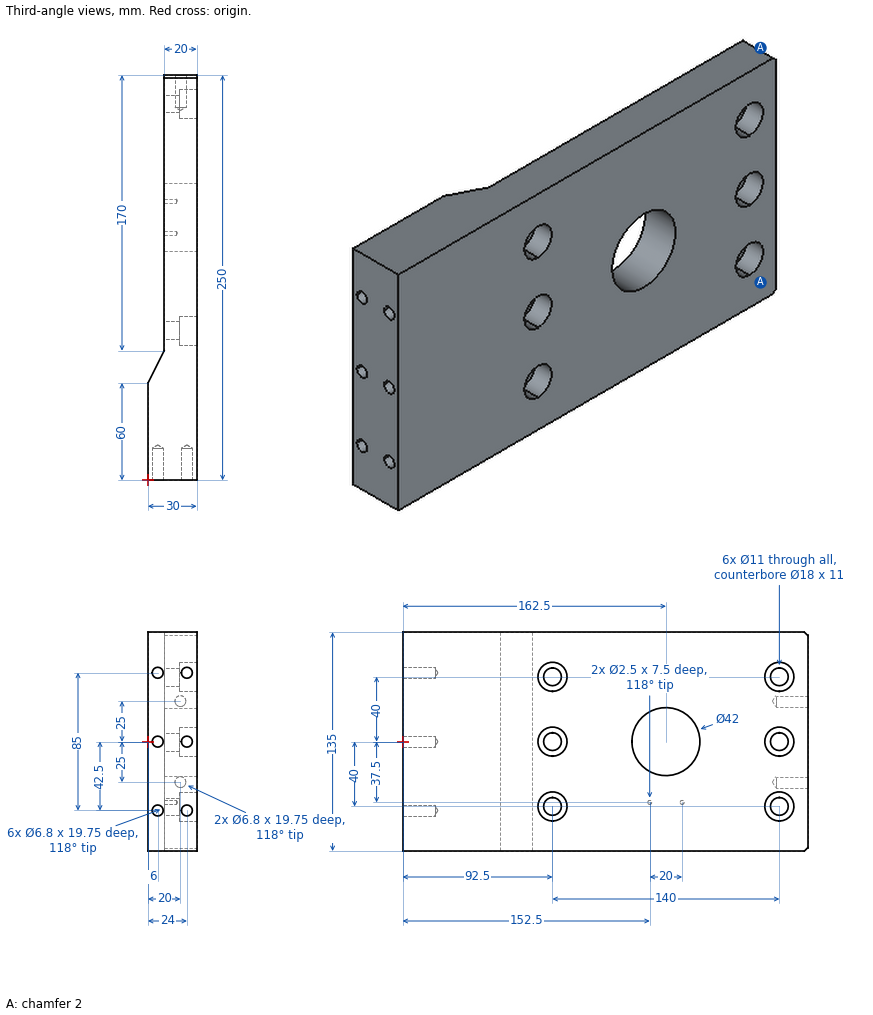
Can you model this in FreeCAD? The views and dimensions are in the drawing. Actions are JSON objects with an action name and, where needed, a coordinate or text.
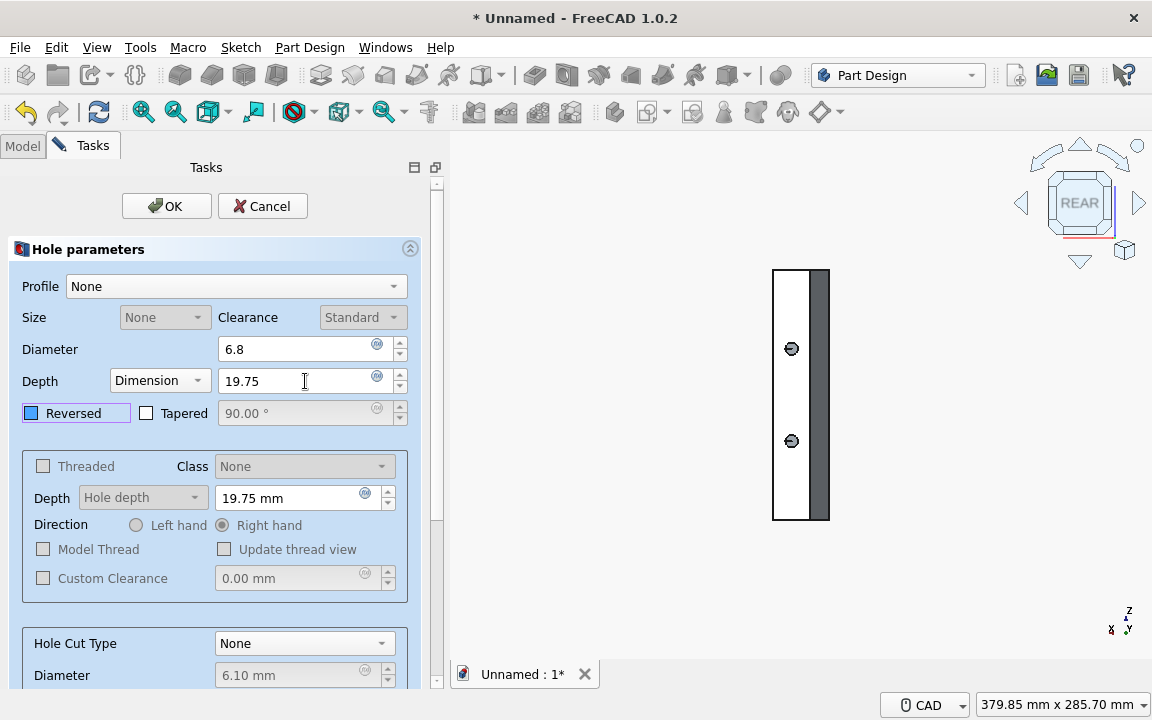
{"action": "left_click", "coordinate": [167, 206]}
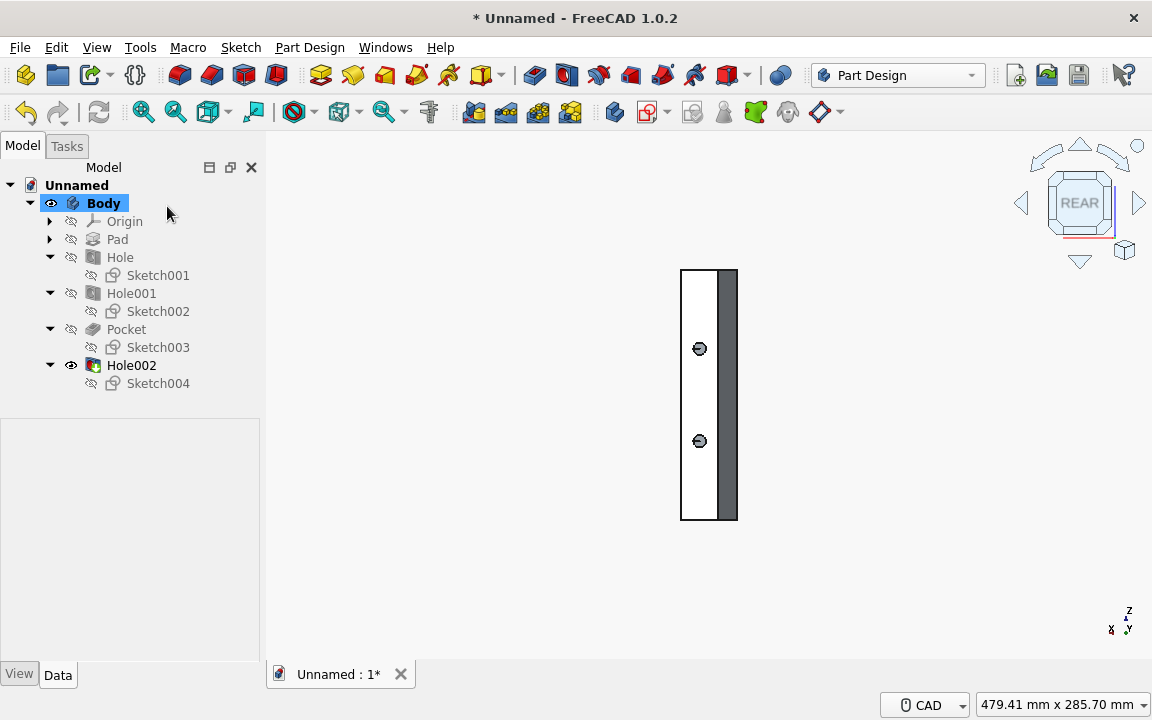
{"action": "left_click", "coordinate": [700, 269]}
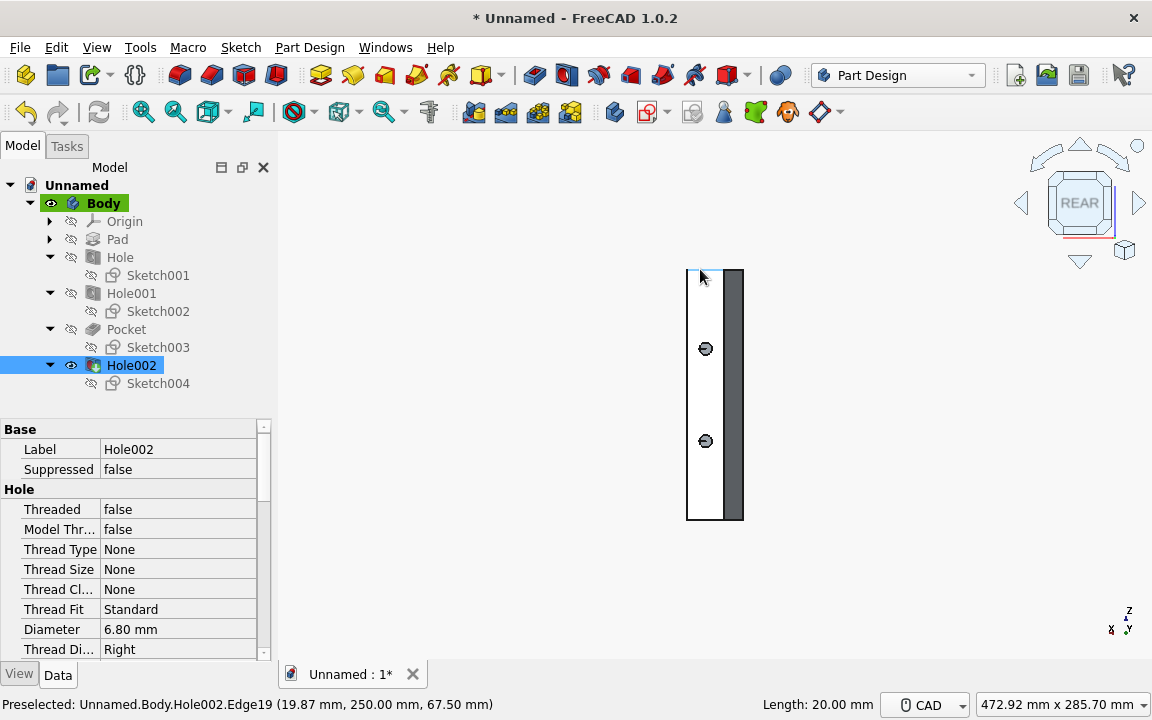
{"action": "left_click", "coordinate": [706, 519], "text": "ctrl"}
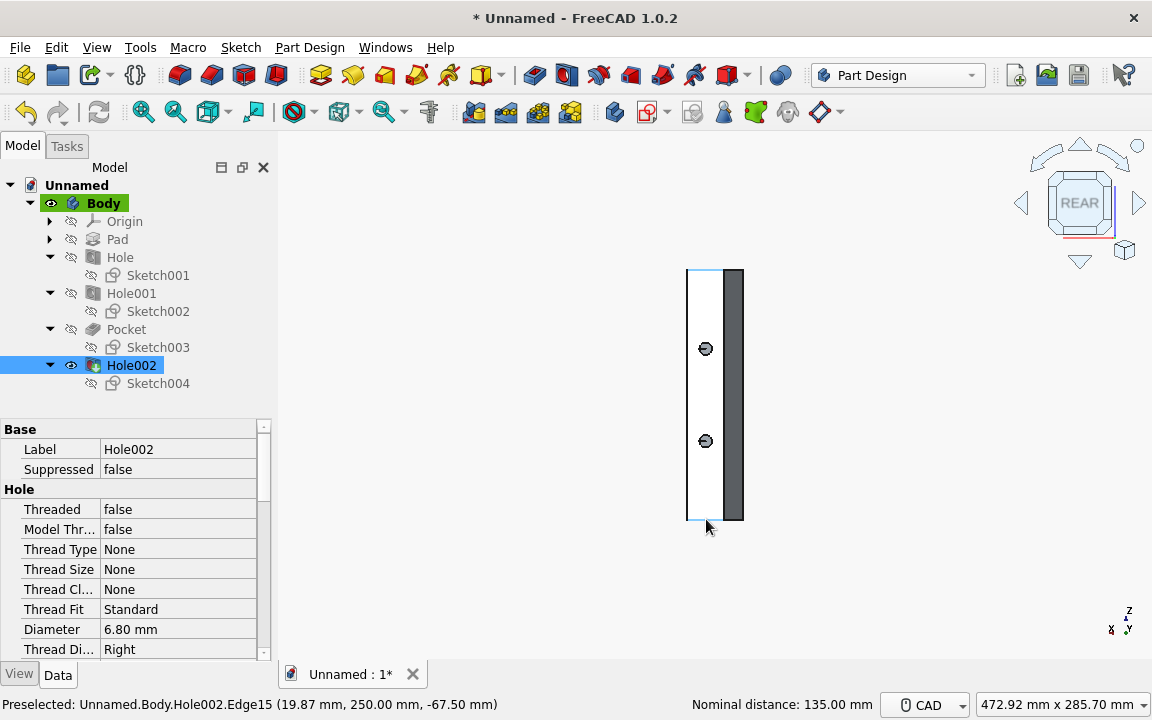
{"action": "left_click", "coordinate": [212, 76]}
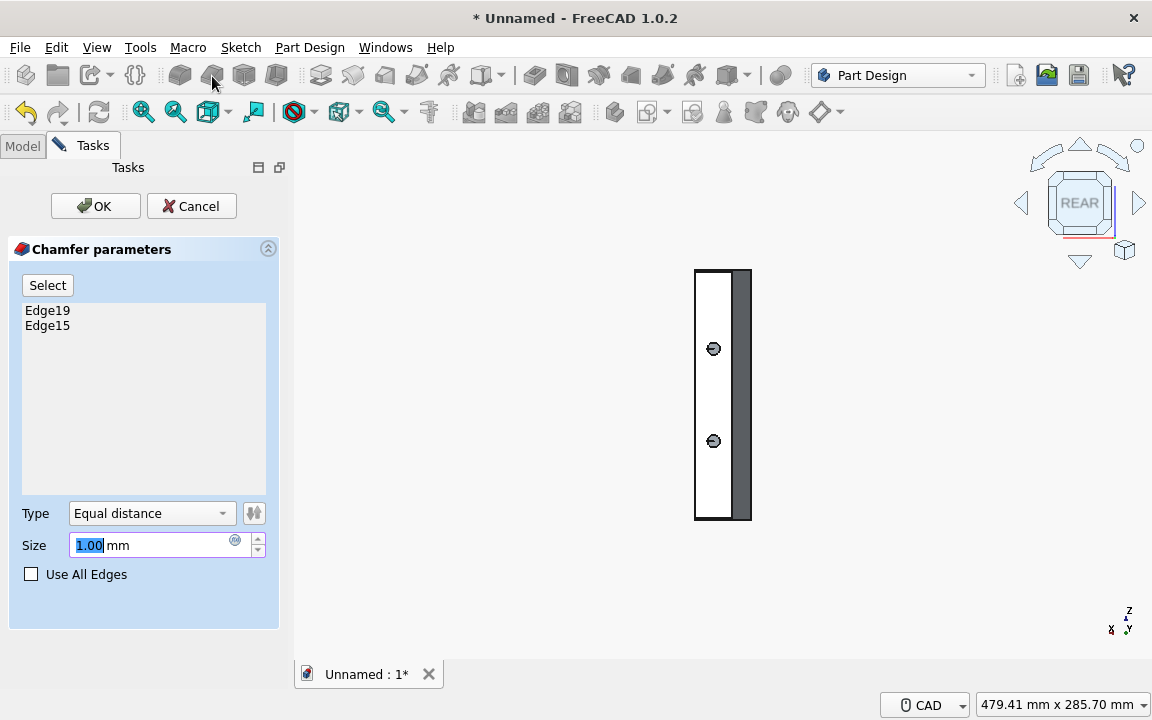
{"action": "type", "text": "2"}
{"action": "key", "text": "Tab"}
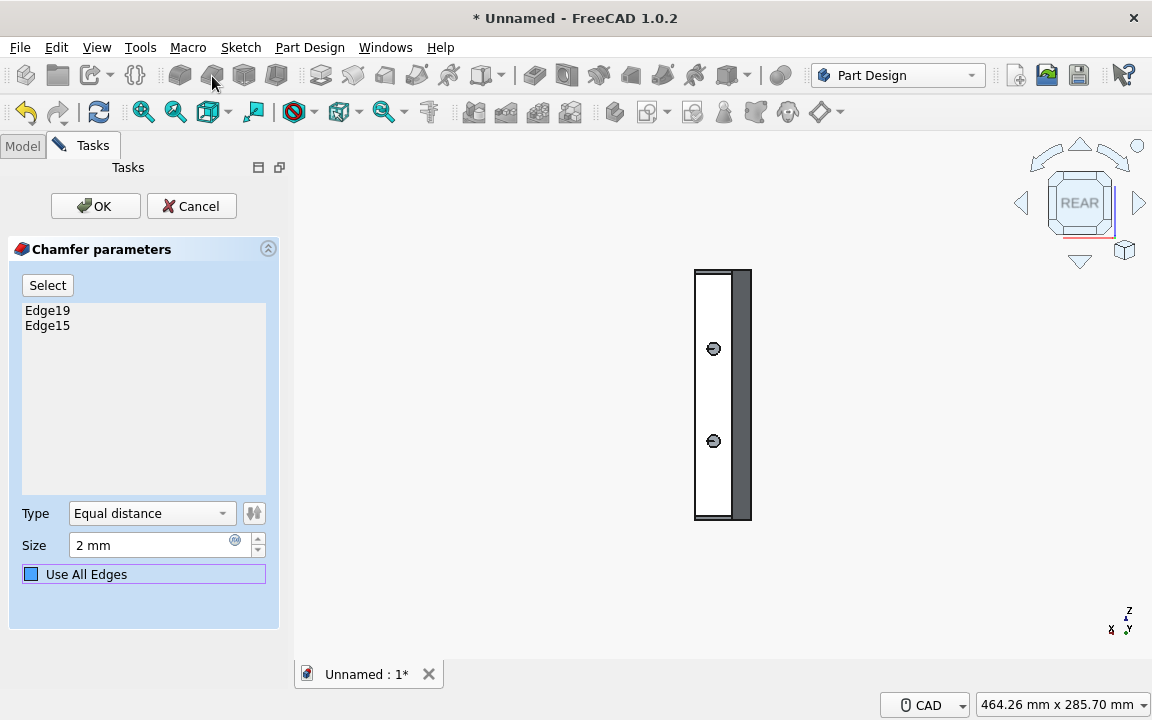
{"action": "left_click", "coordinate": [96, 206]}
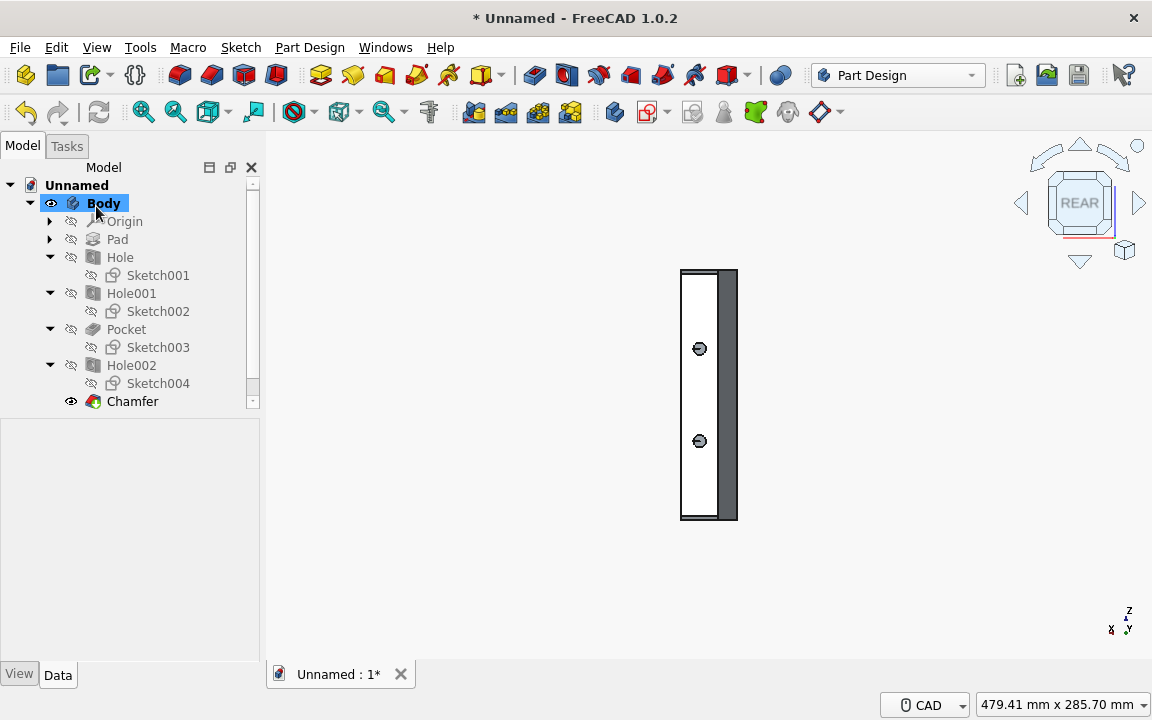
{"action": "key", "text": "6"}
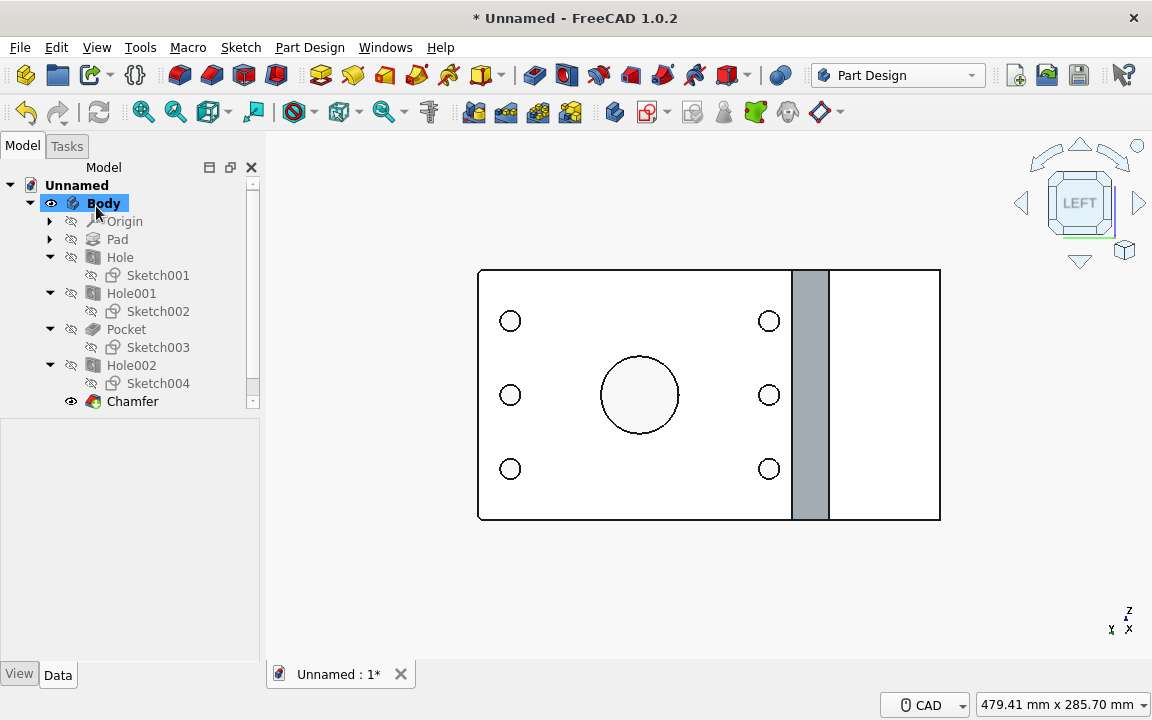
{"action": "left_click", "coordinate": [590, 323]}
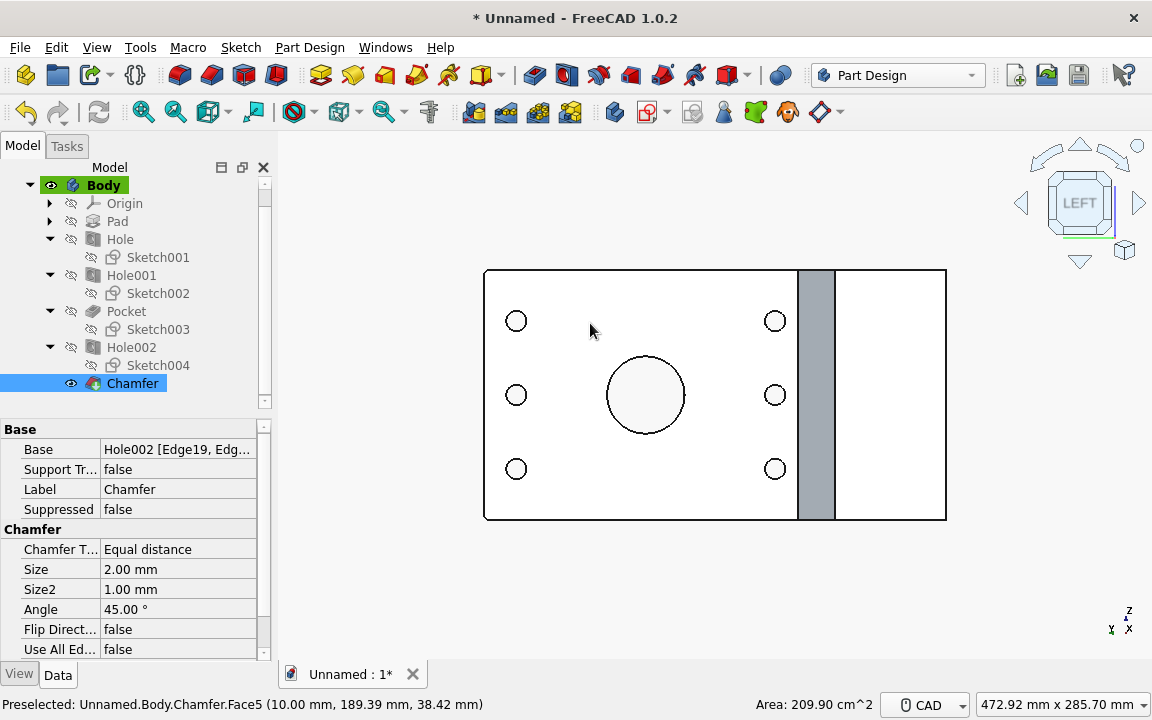
{"action": "left_click", "coordinate": [648, 112]}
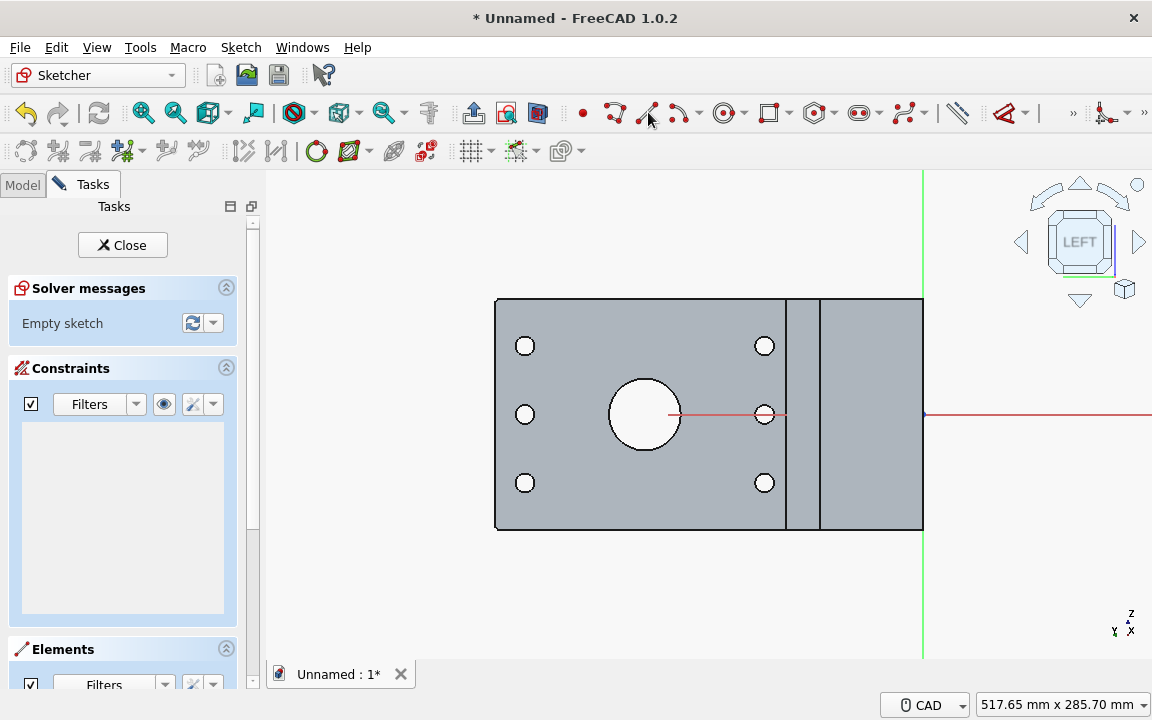
{"action": "left_click", "coordinate": [538, 114]}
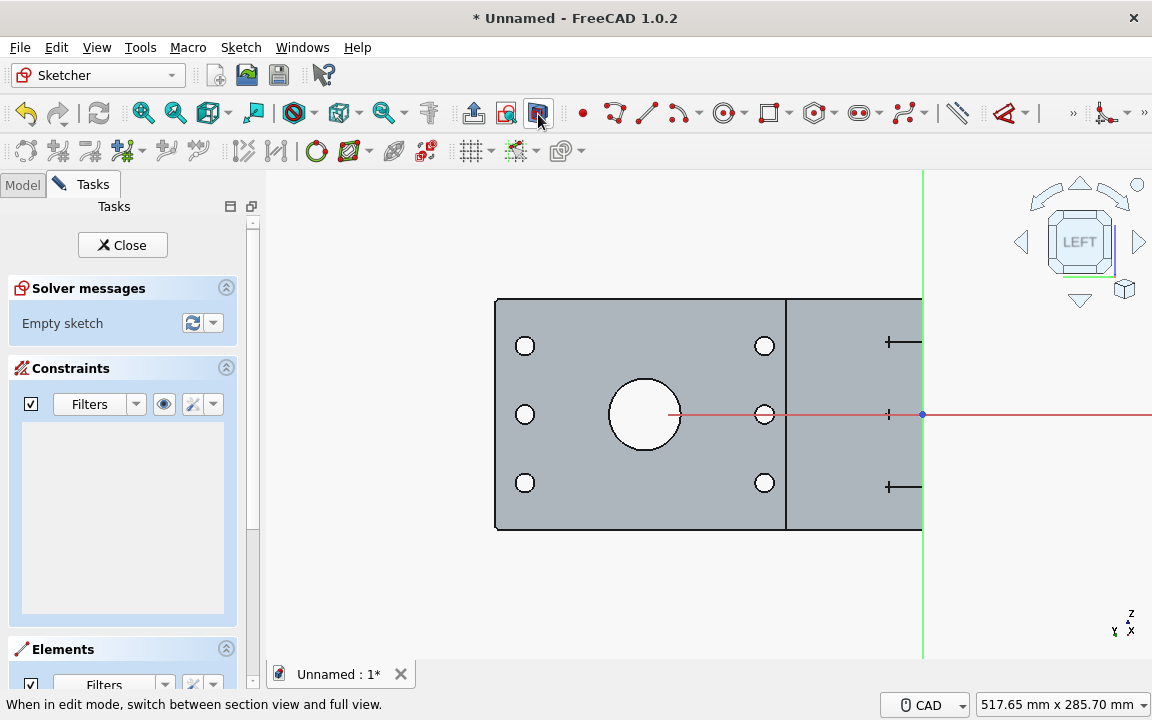
{"action": "scroll", "coordinate": [645, 484], "scroll_direction": "up", "scroll_amount": 13}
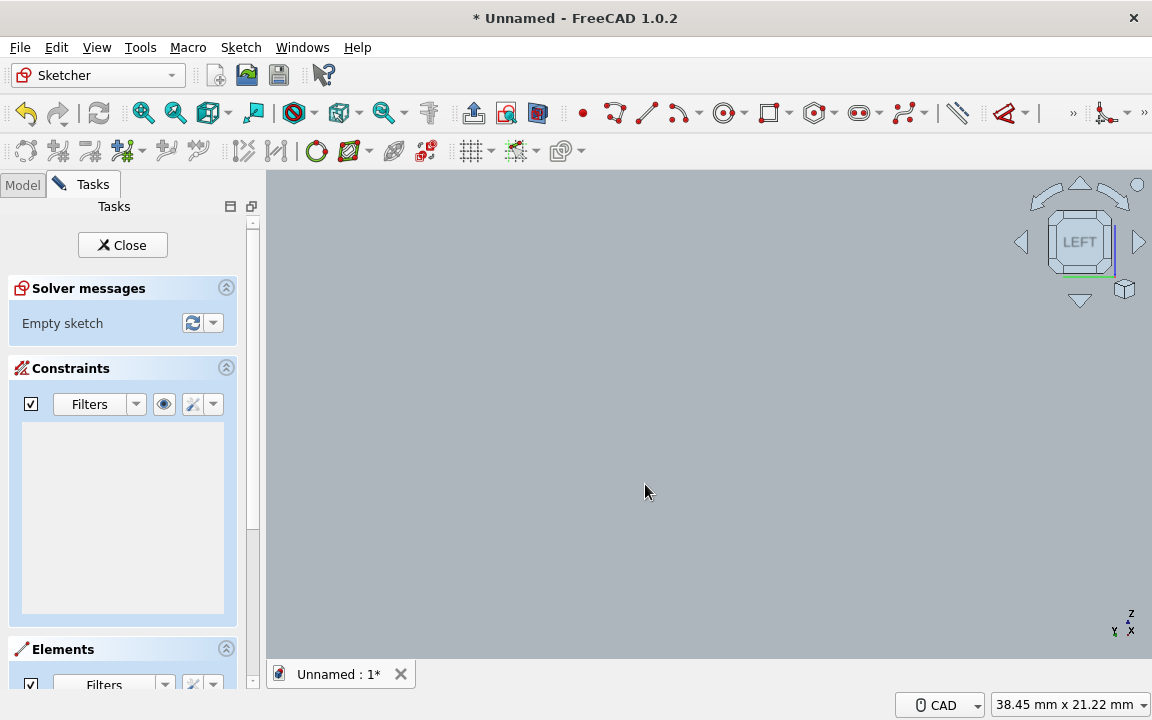
{"action": "left_click", "coordinate": [724, 114]}